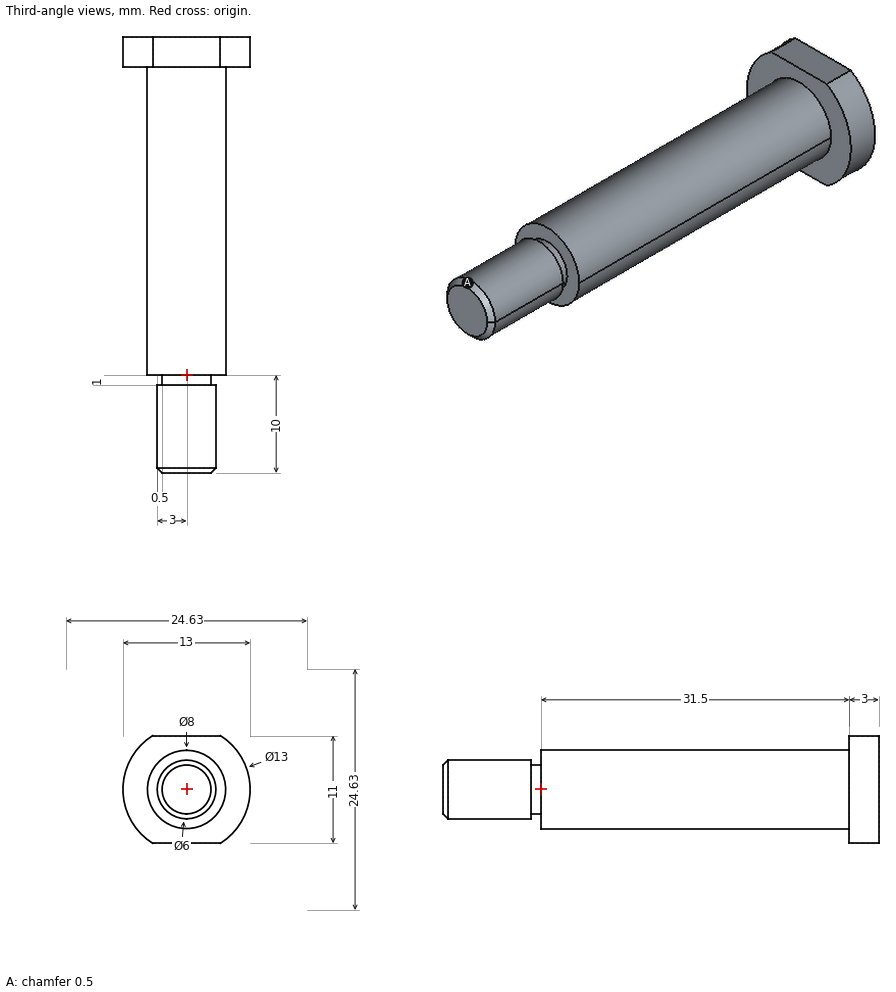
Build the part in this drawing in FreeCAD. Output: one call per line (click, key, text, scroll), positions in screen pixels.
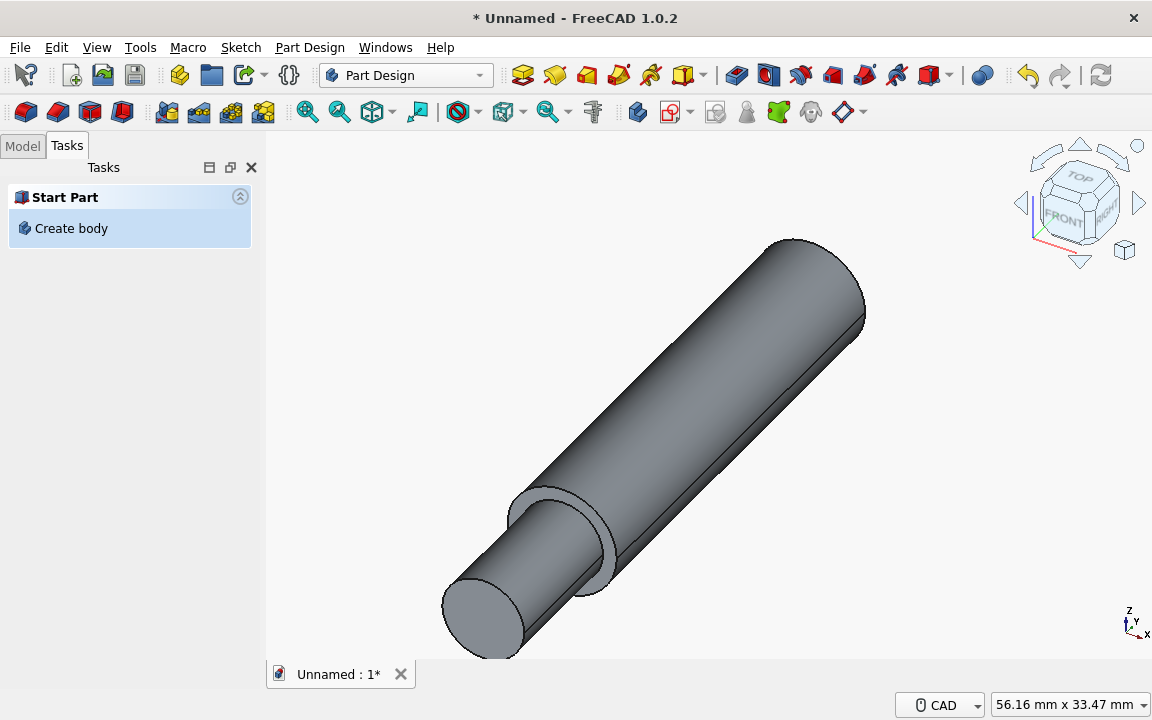
key(v)
key(f)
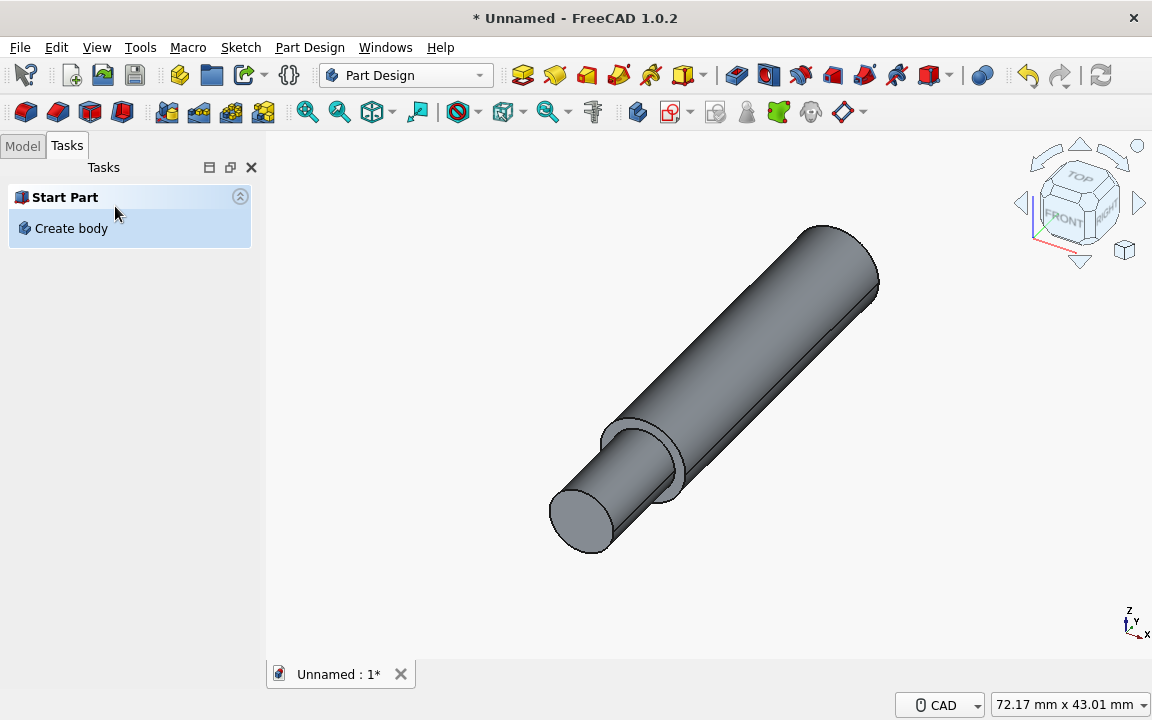
key(4)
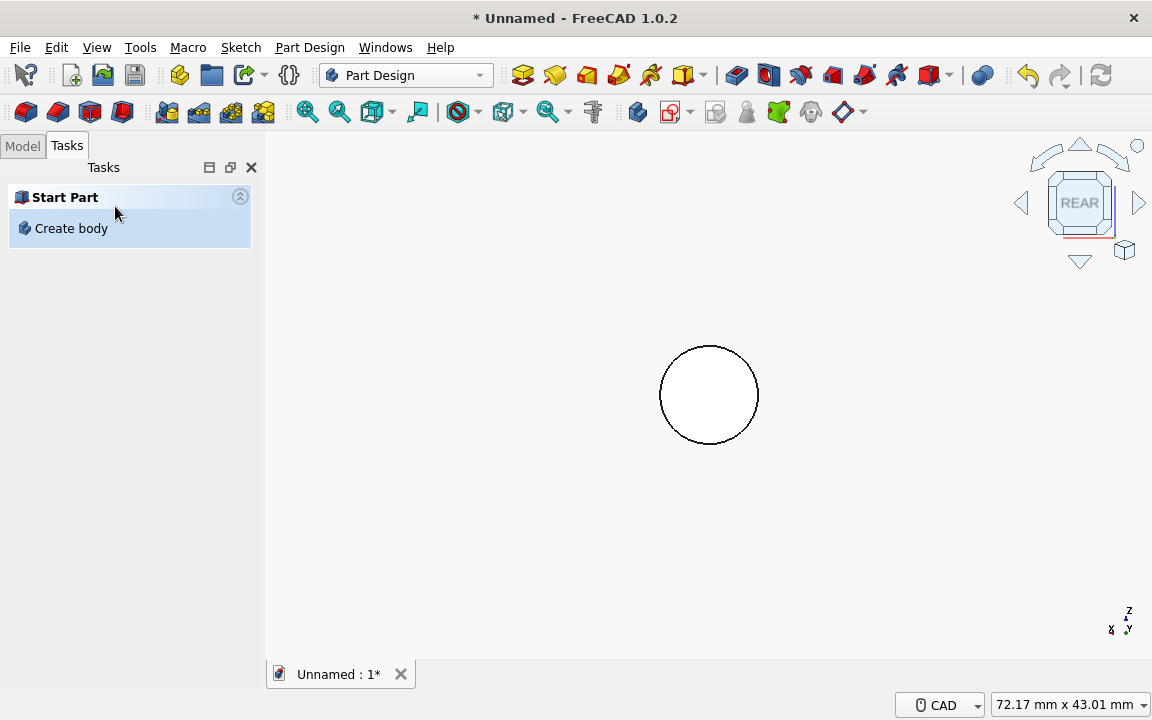
key(v)
key(f)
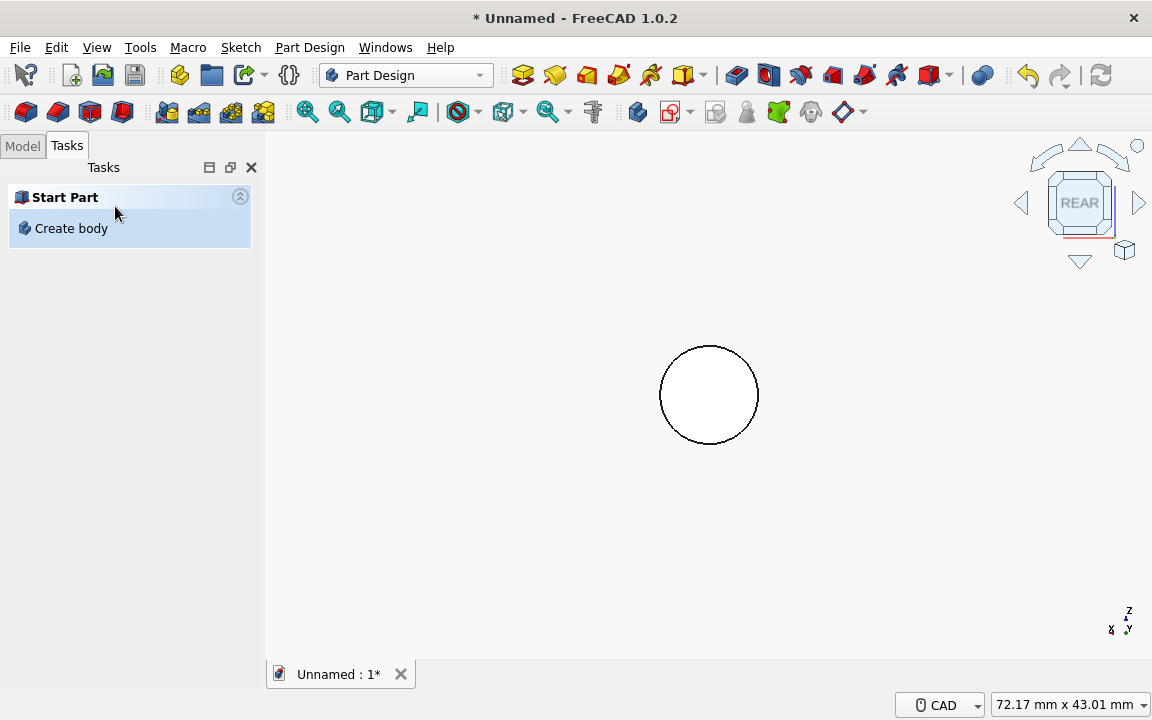
click(709, 394)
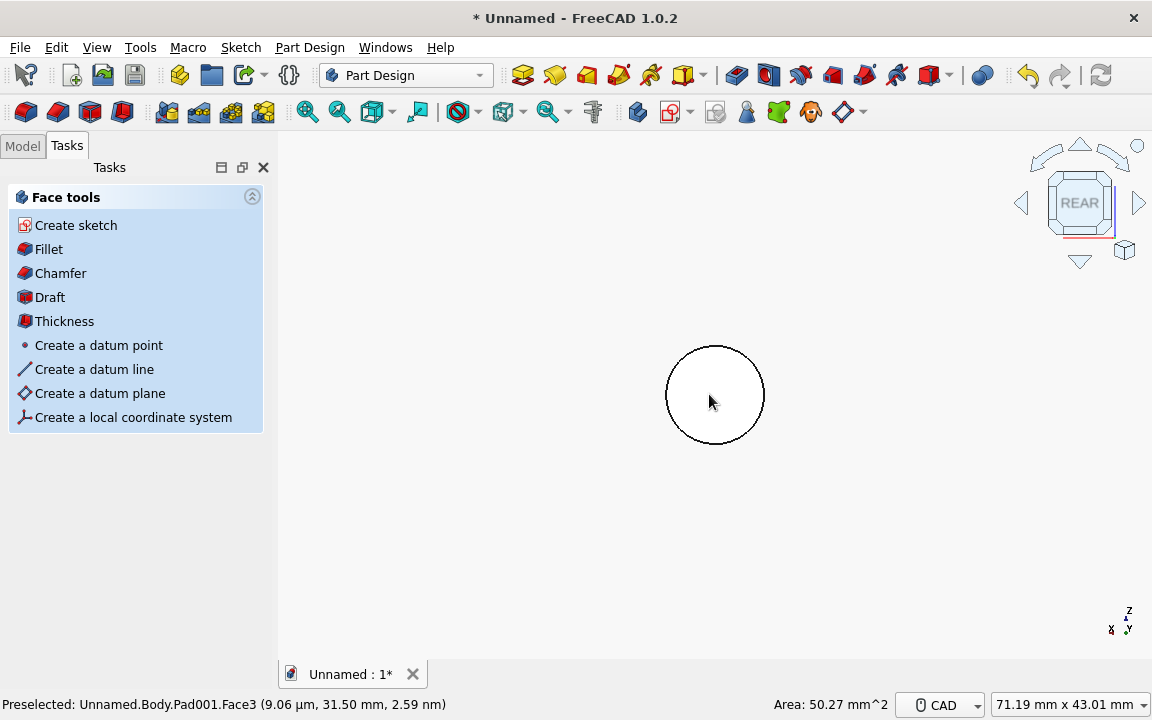
click(670, 112)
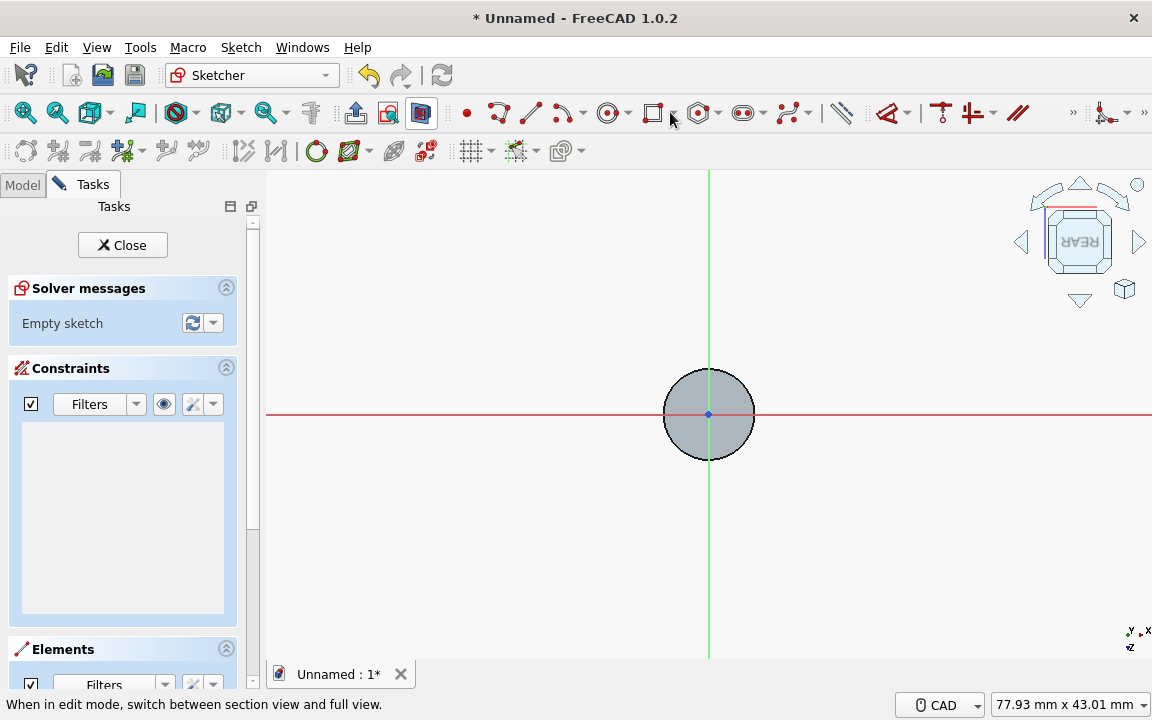
scroll(765, 414, up, 4)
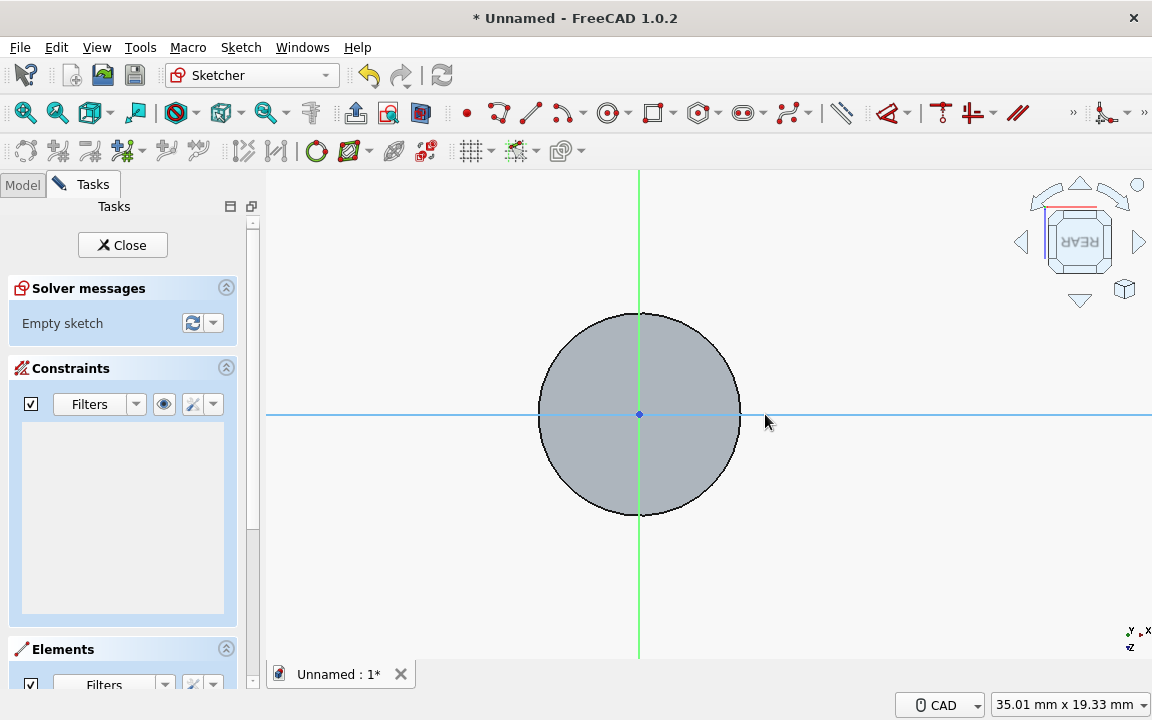
click(608, 114)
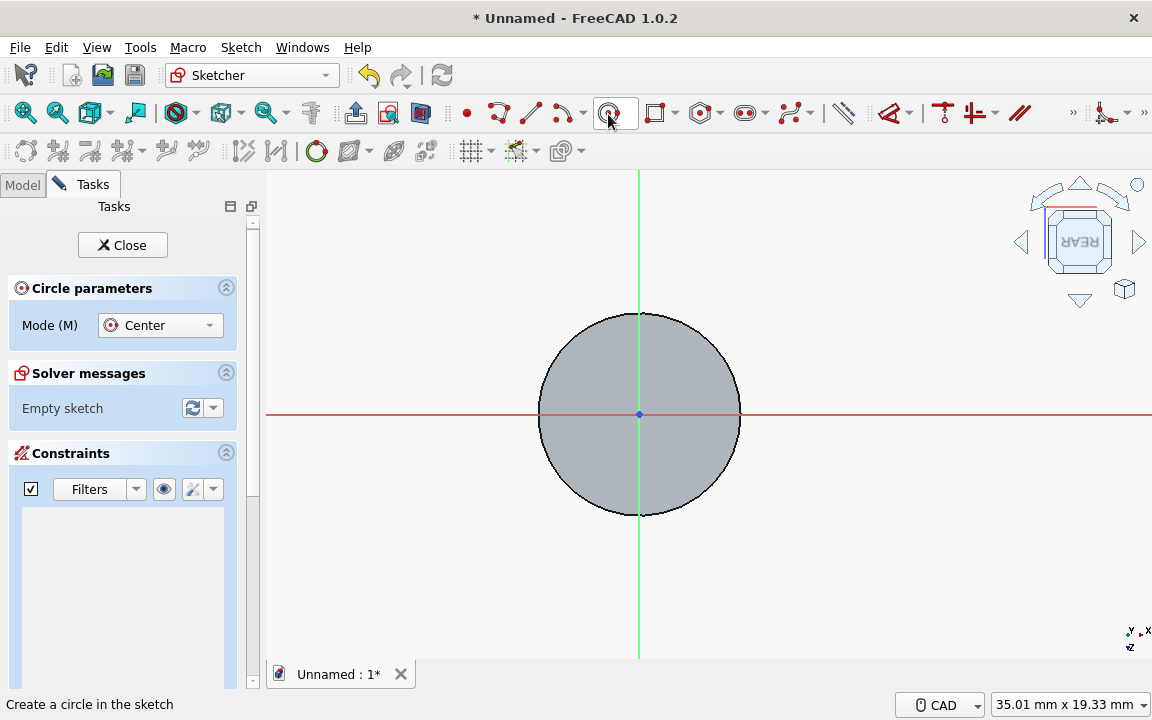
click(639, 414)
move(756, 298)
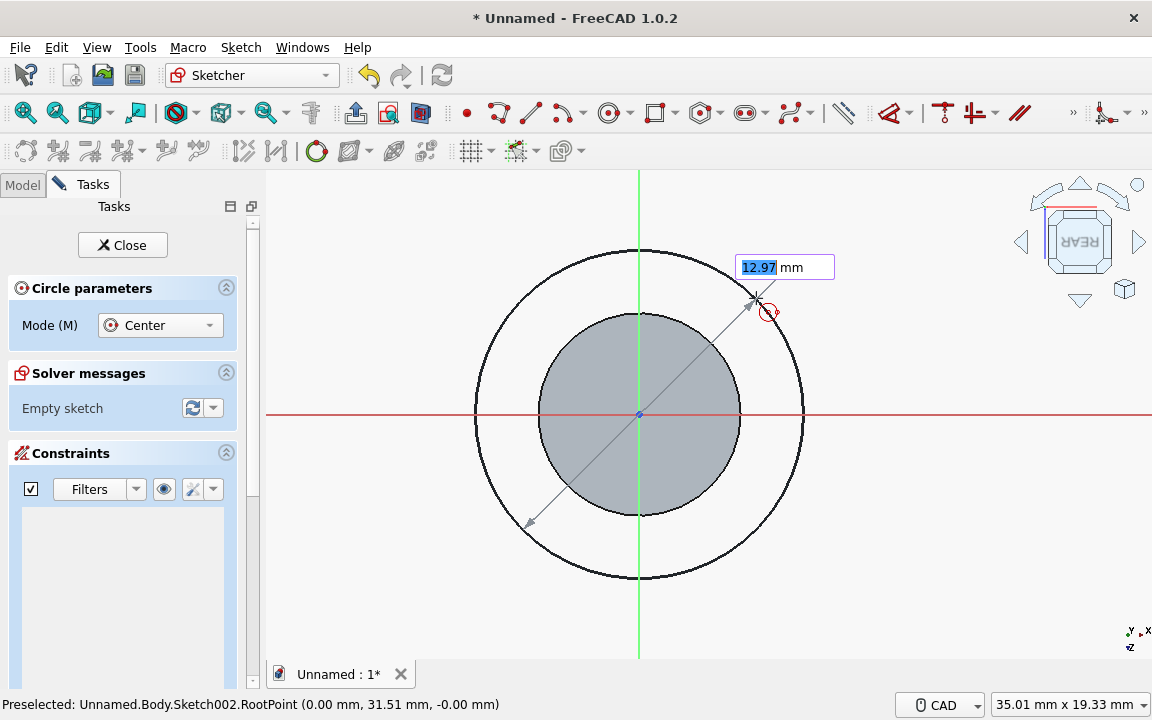
text(13)
key(Return)
key(Escape)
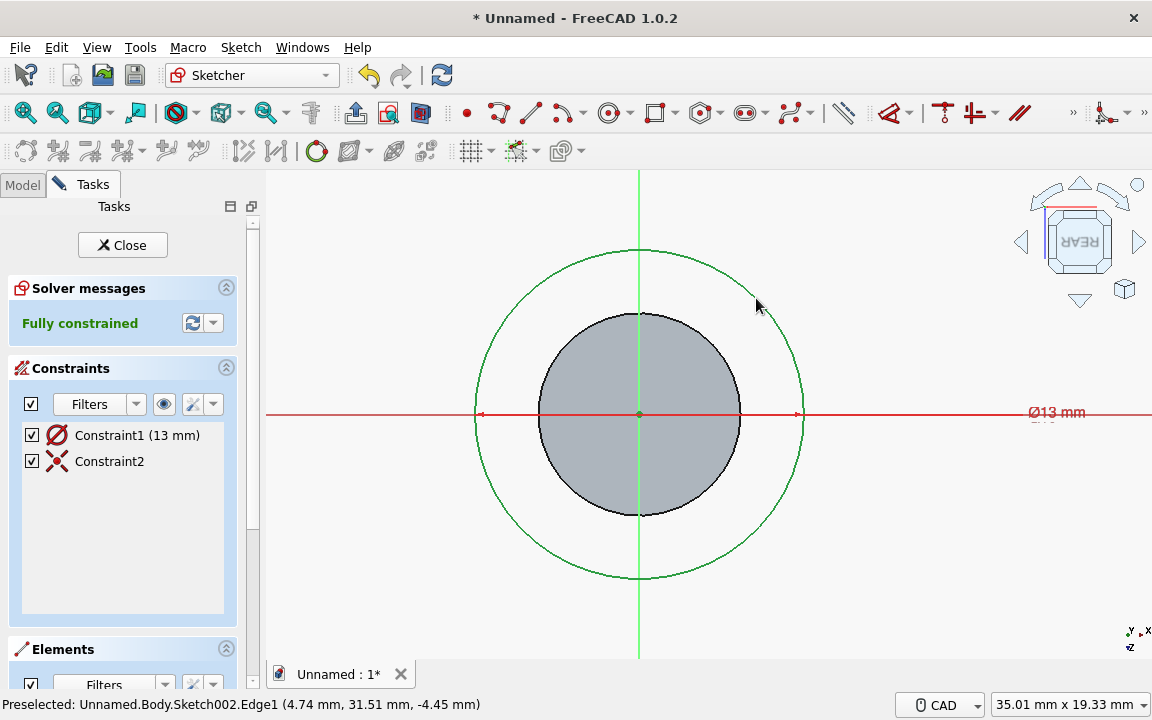
click(123, 245)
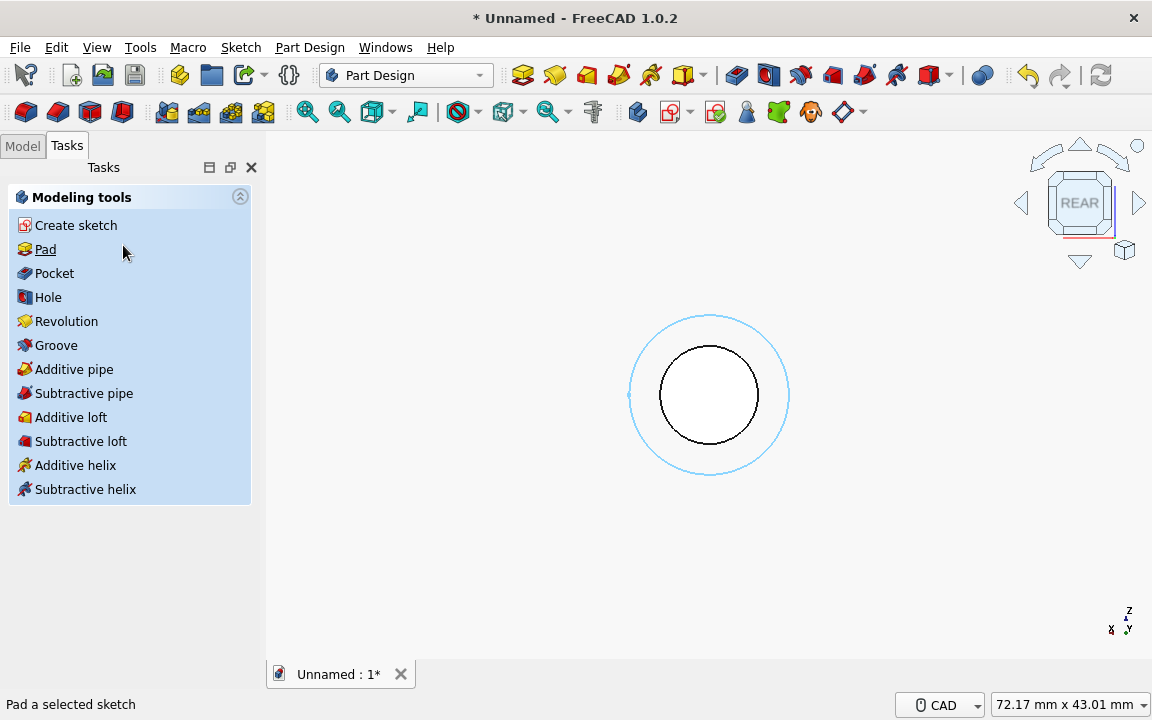
click(524, 76)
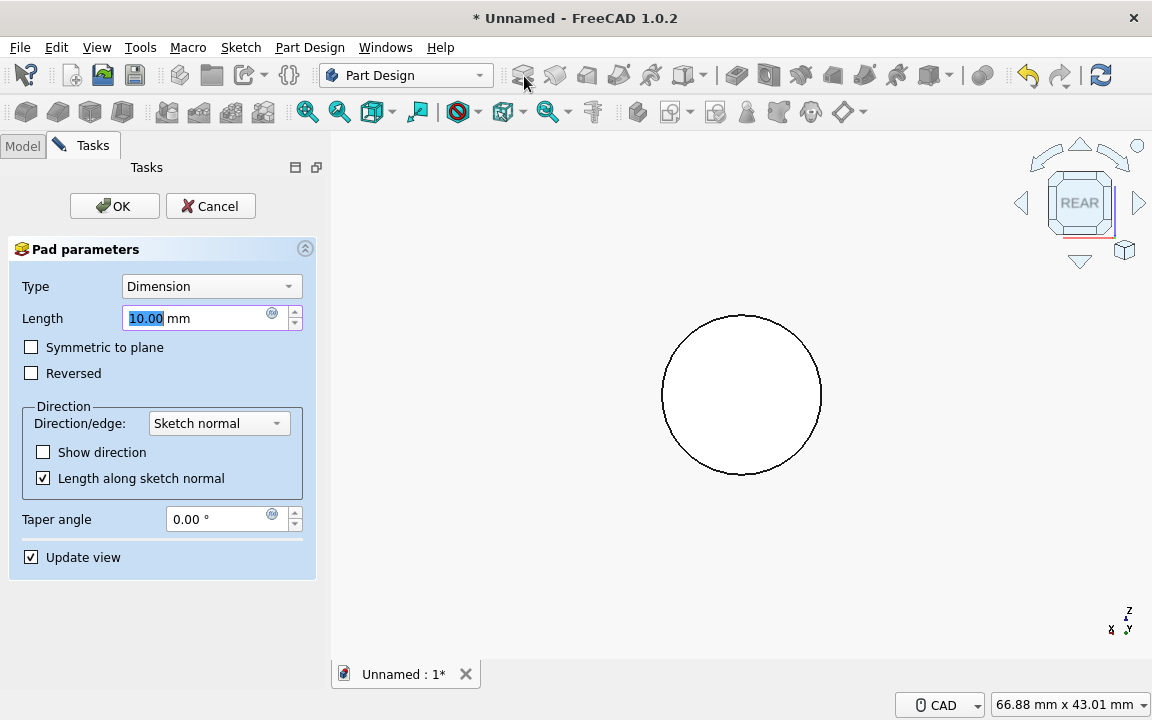
text(3)
key(Tab)